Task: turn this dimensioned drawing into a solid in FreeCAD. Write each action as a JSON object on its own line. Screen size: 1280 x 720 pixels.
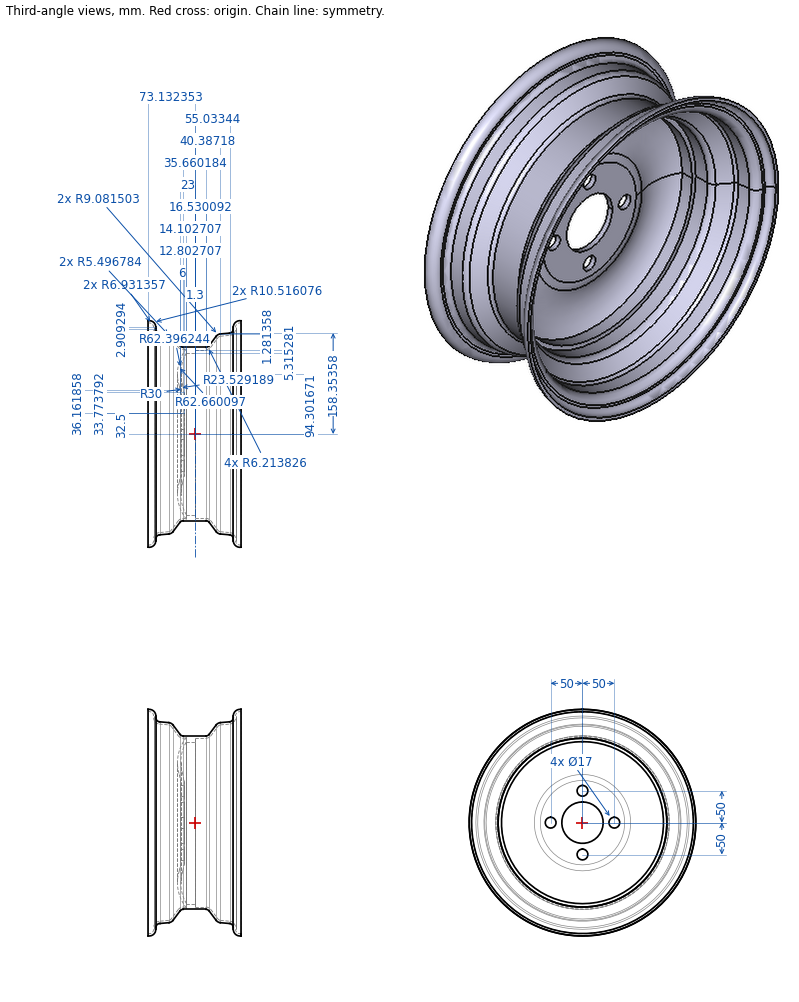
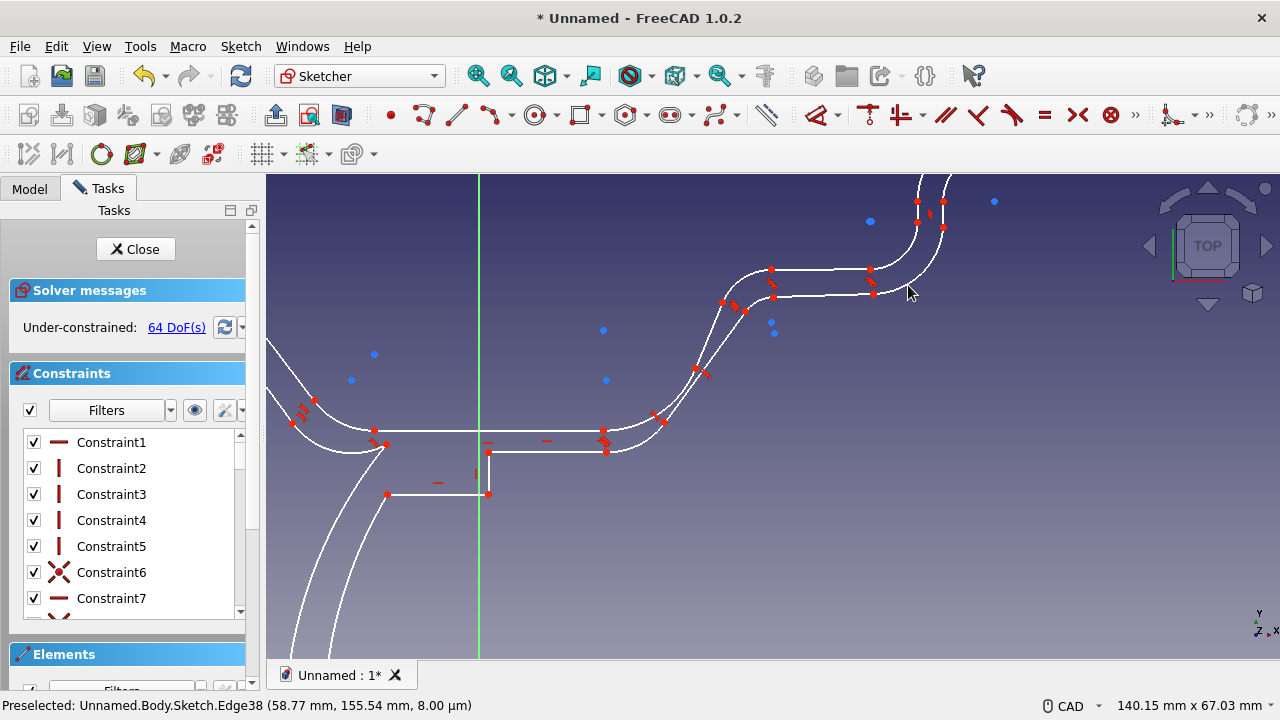
{"action": "scroll", "coordinate": [943, 217], "scroll_direction": "up", "scroll_amount": 2}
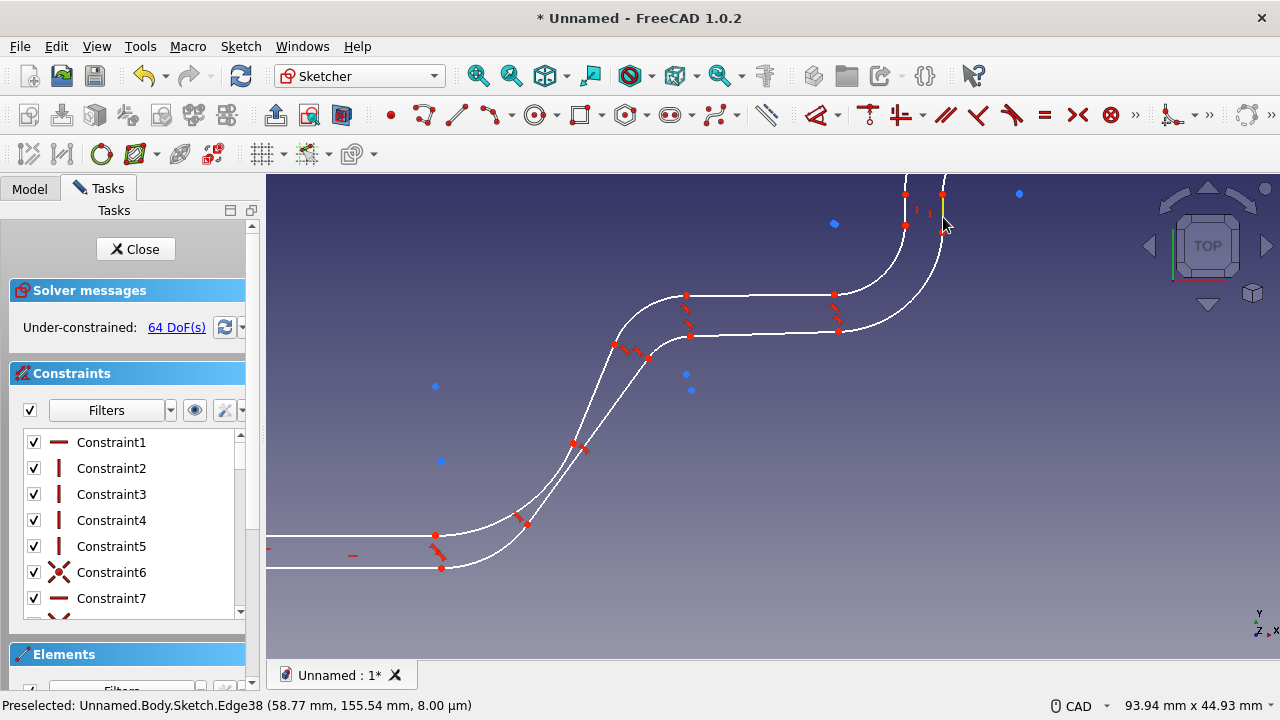
{"action": "left_click", "coordinate": [943, 217]}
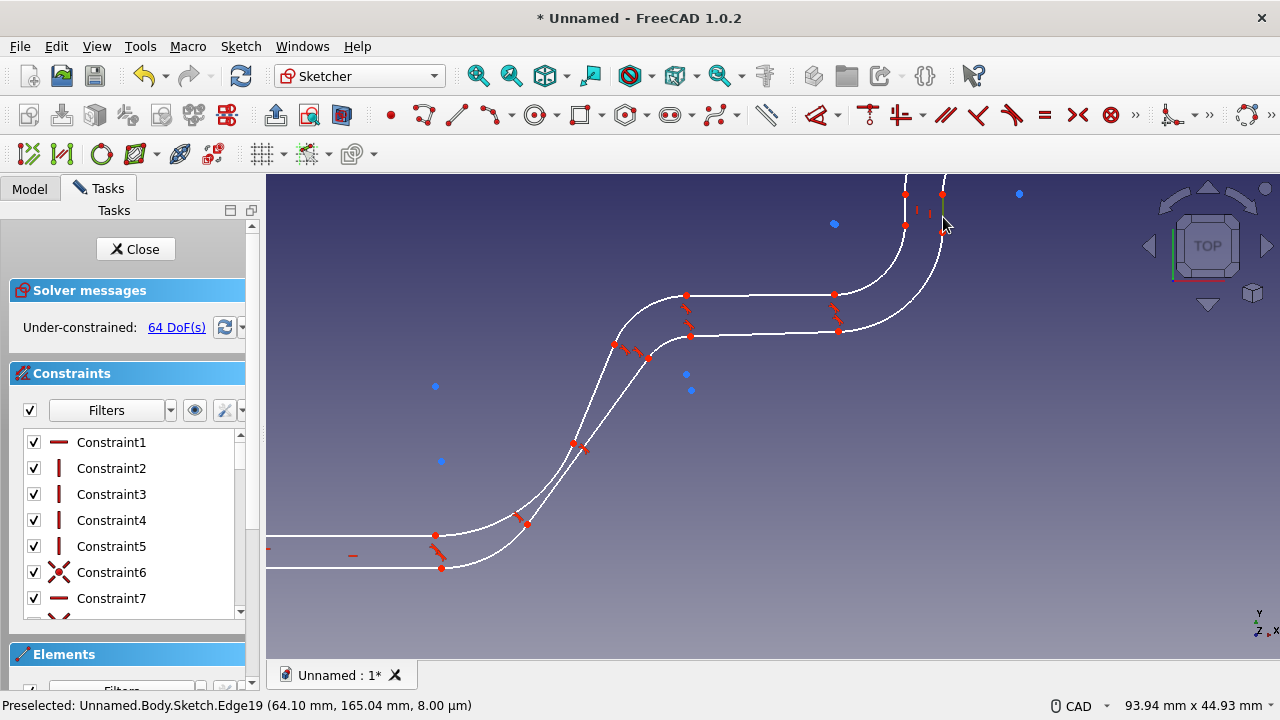
{"action": "left_click", "coordinate": [884, 320]}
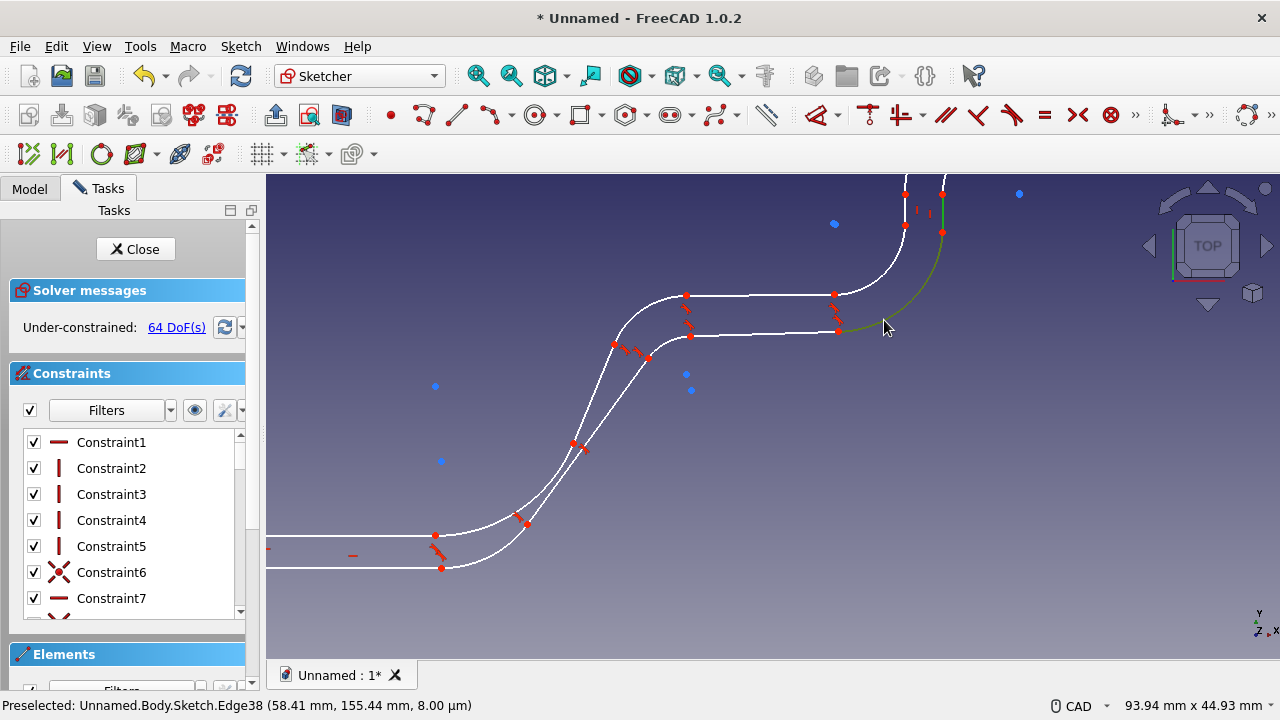
{"action": "key", "text": "t"}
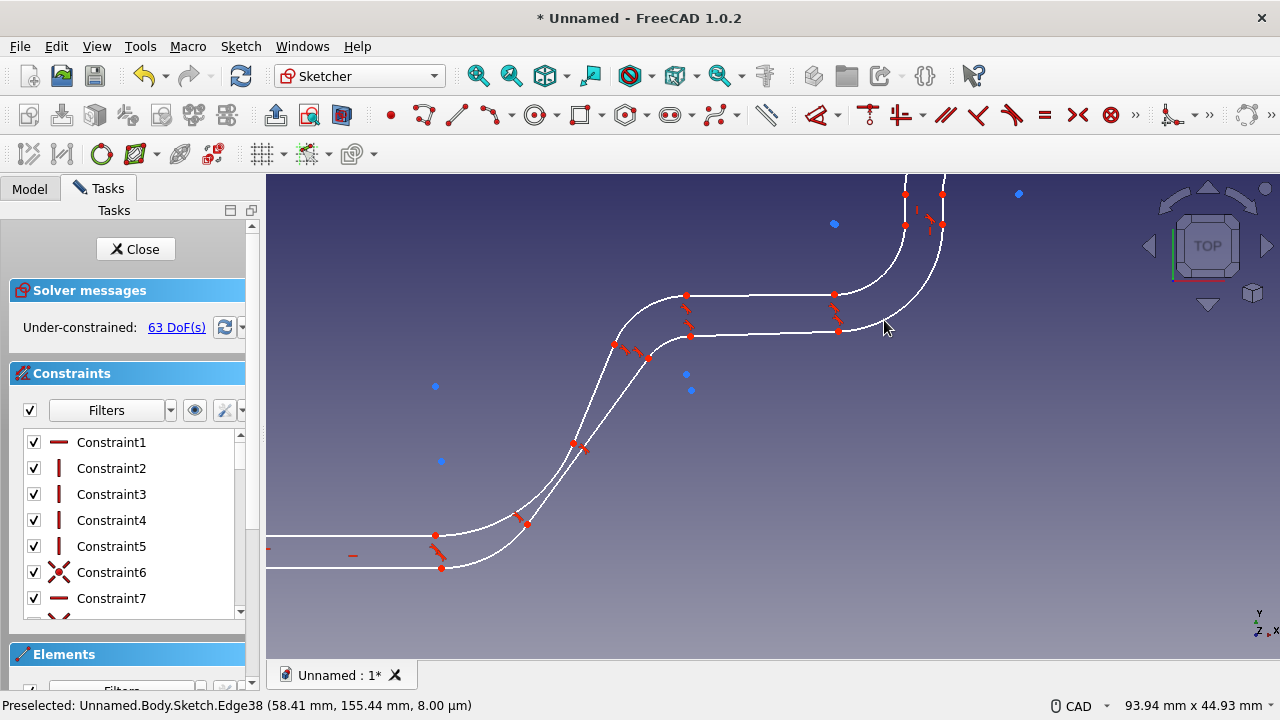
{"action": "left_click", "coordinate": [943, 212]}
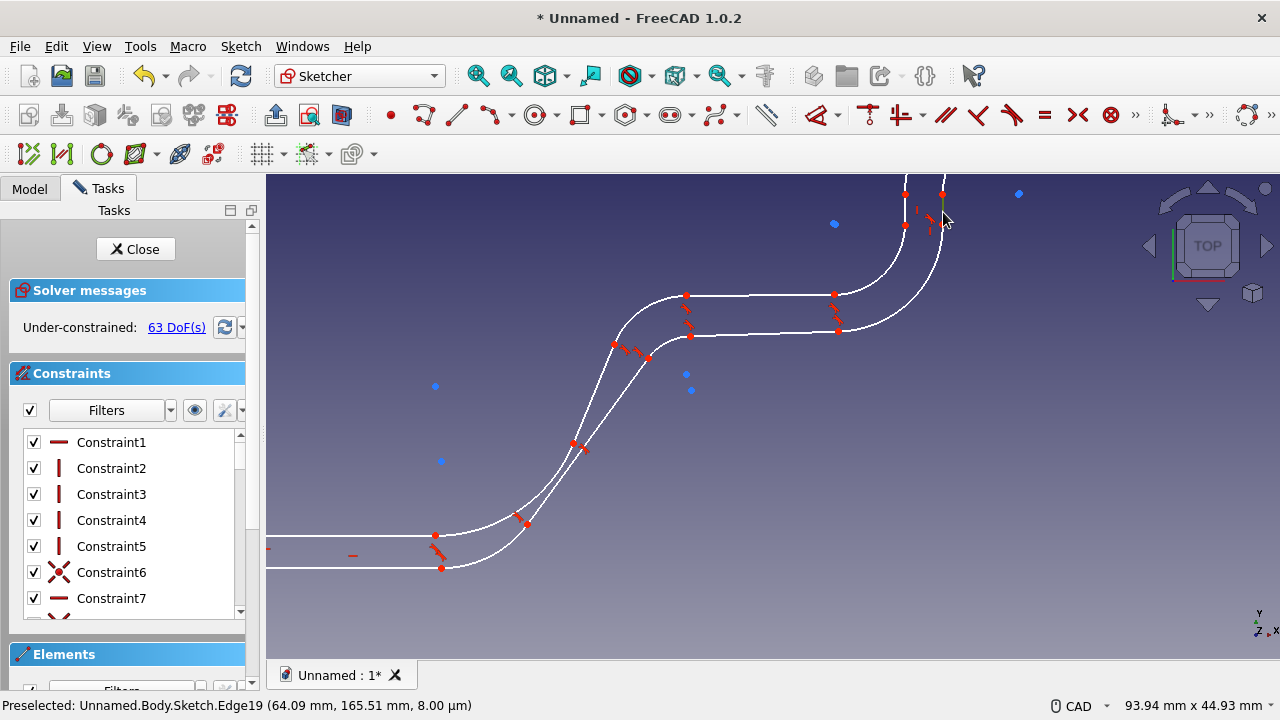
{"action": "scroll", "coordinate": [794, 293], "scroll_direction": "down", "scroll_amount": 9}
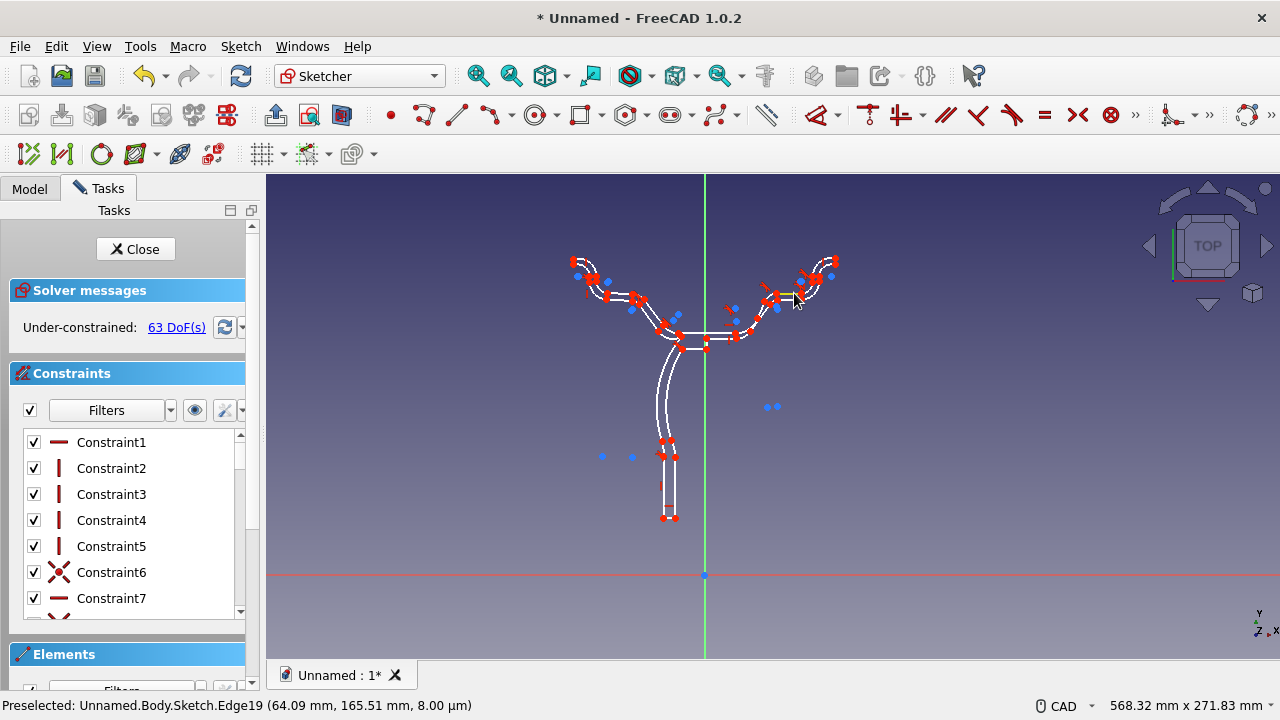
{"action": "scroll", "coordinate": [828, 265], "scroll_direction": "up", "scroll_amount": 4}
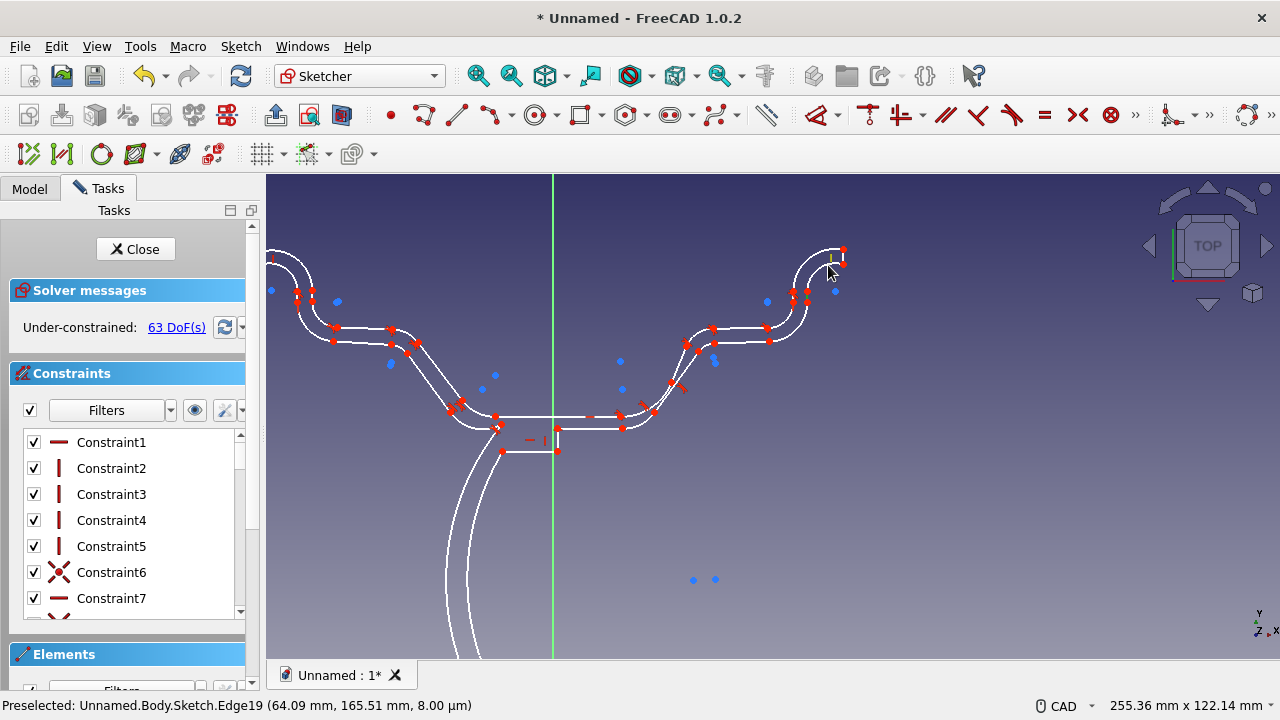
{"action": "left_click", "coordinate": [828, 264]}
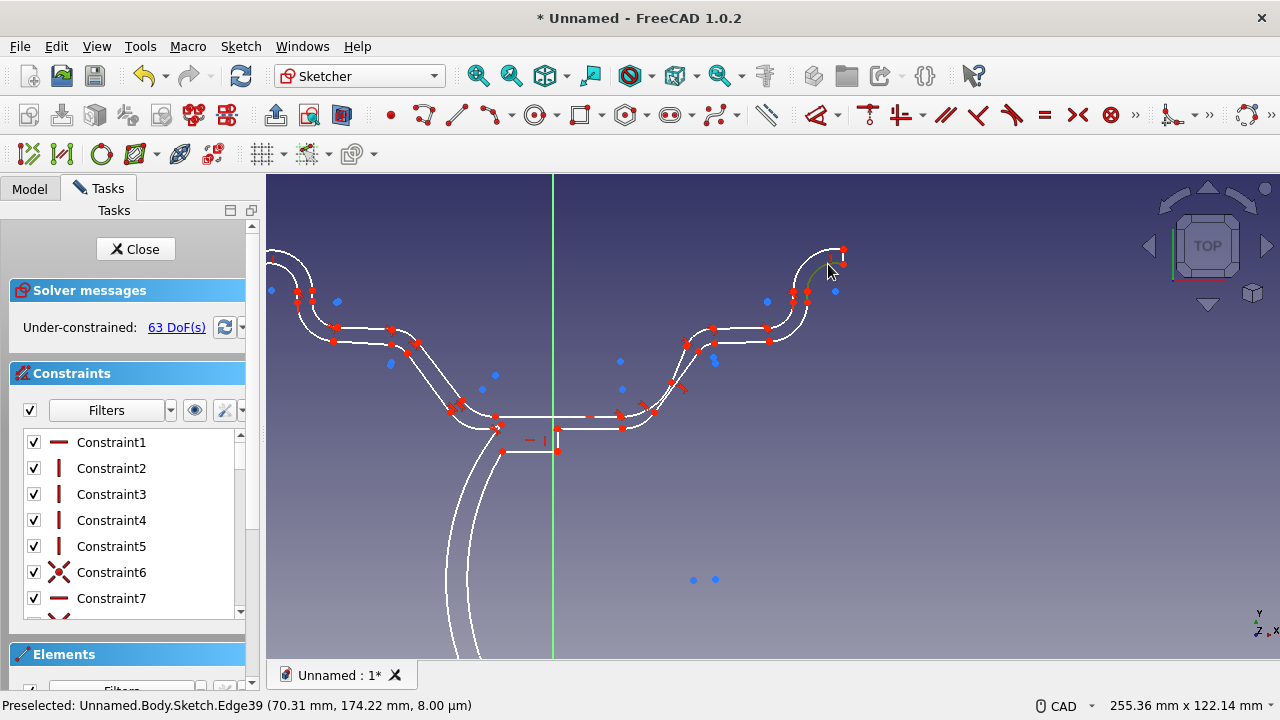
{"action": "key", "text": "t"}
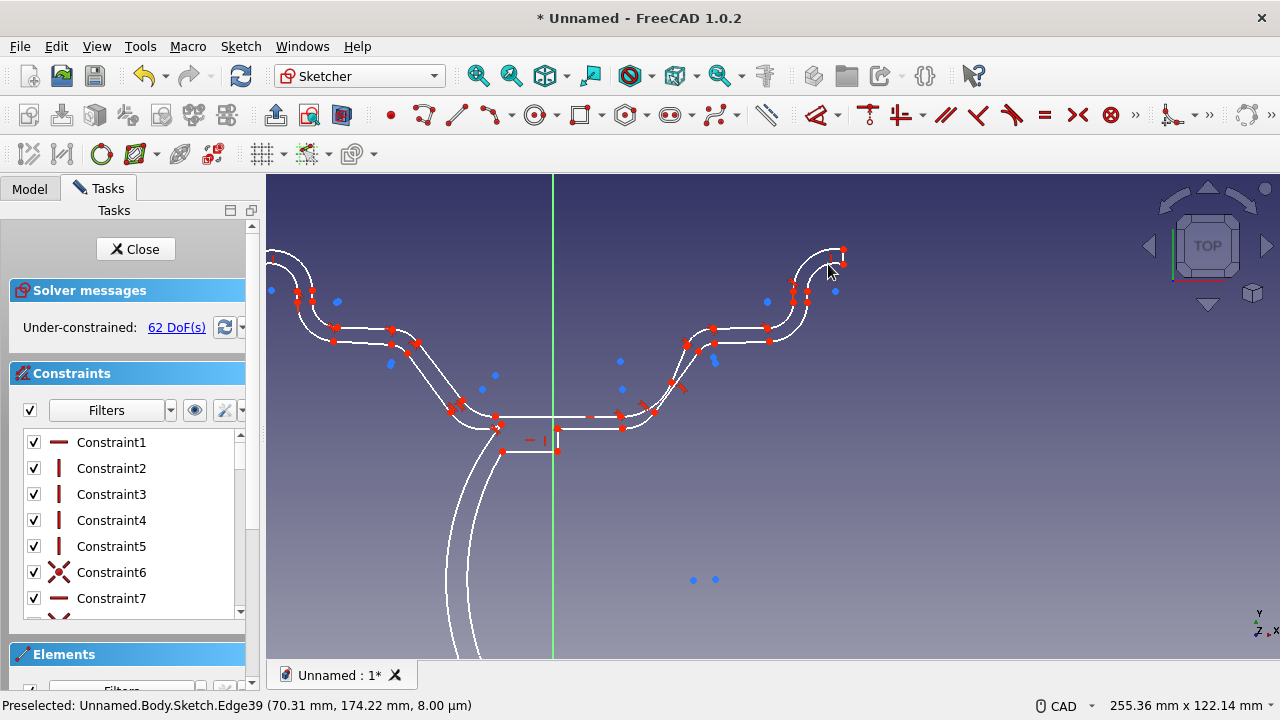
{"action": "scroll", "coordinate": [793, 297], "scroll_direction": "up", "scroll_amount": 5}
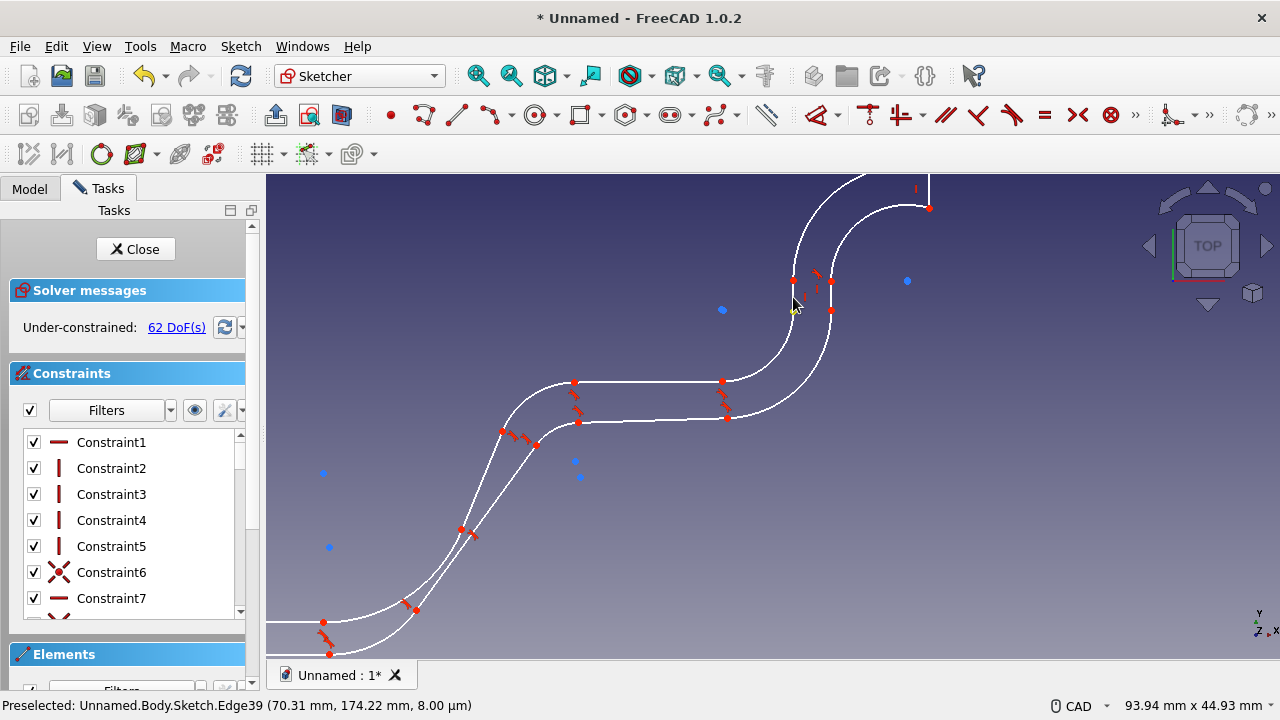
{"action": "left_click", "coordinate": [793, 296]}